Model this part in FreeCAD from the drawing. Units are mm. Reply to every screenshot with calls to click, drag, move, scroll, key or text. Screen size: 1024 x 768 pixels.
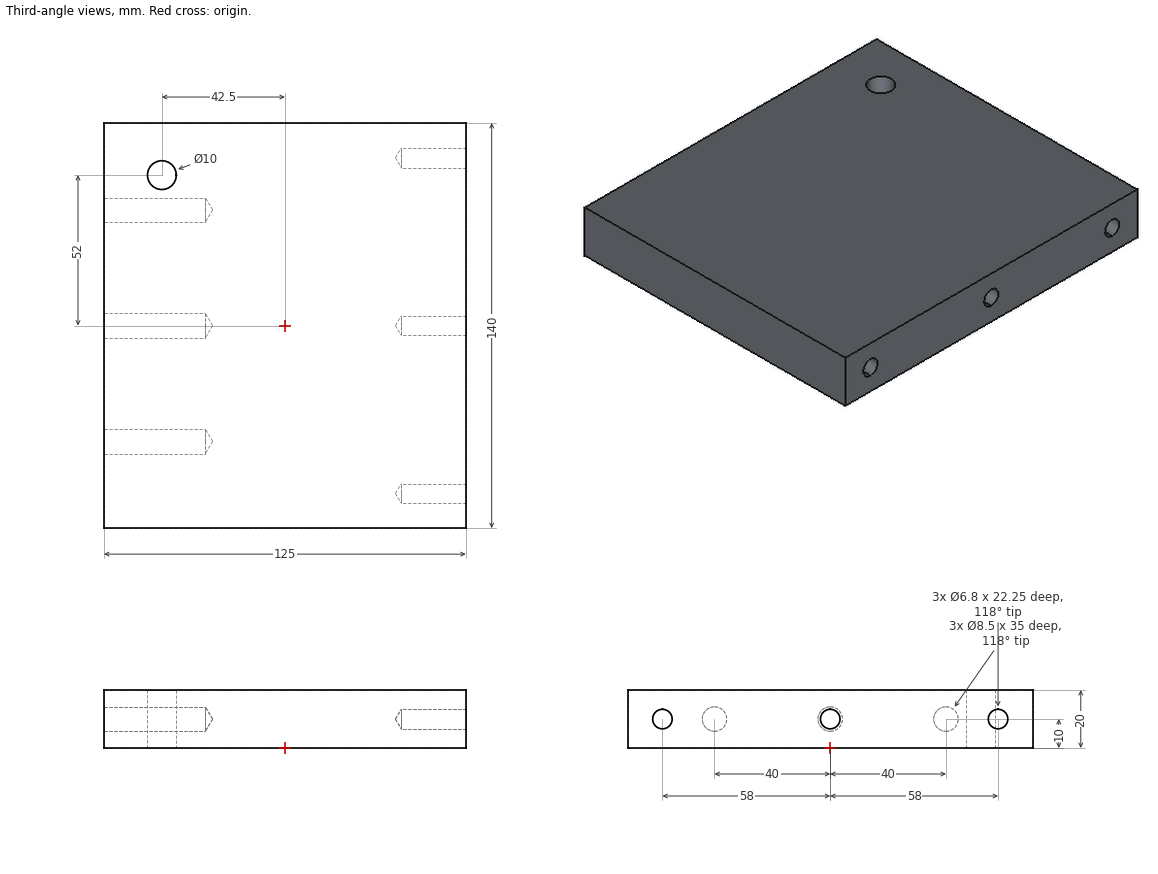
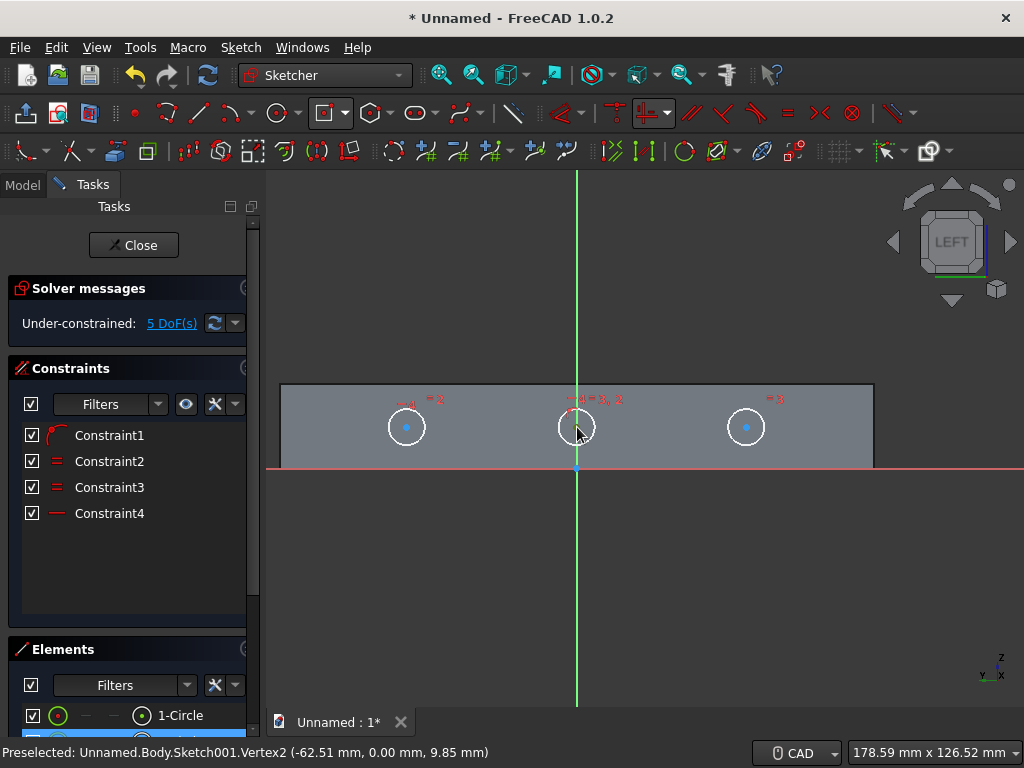
click(746, 427)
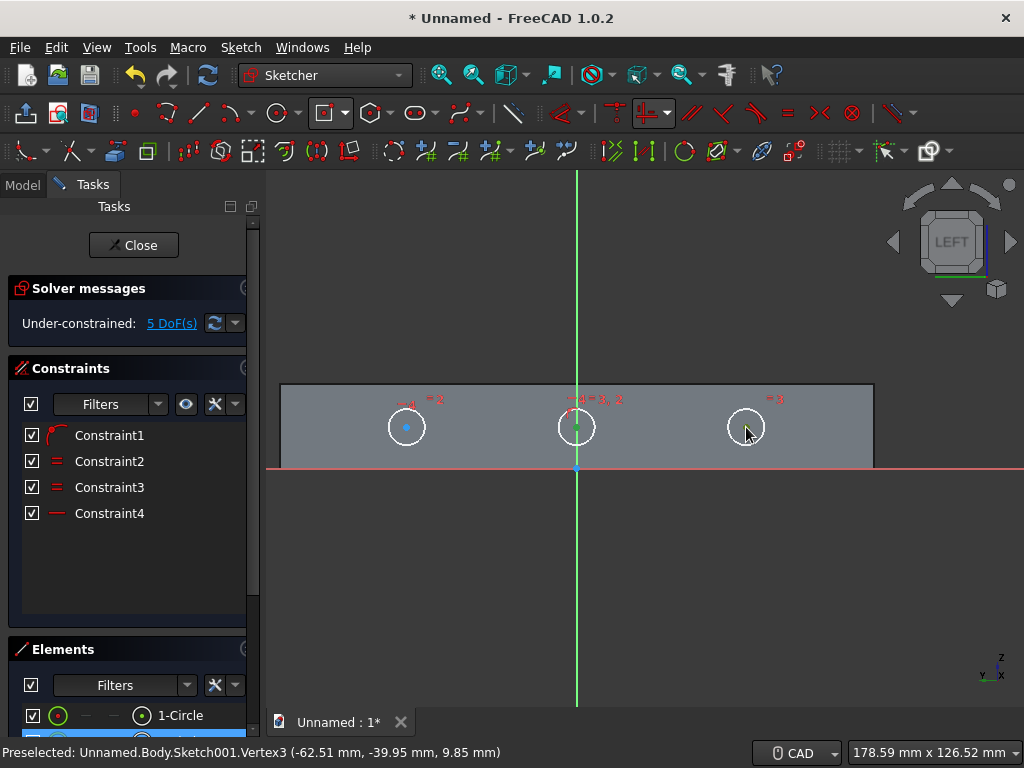
click(670, 114)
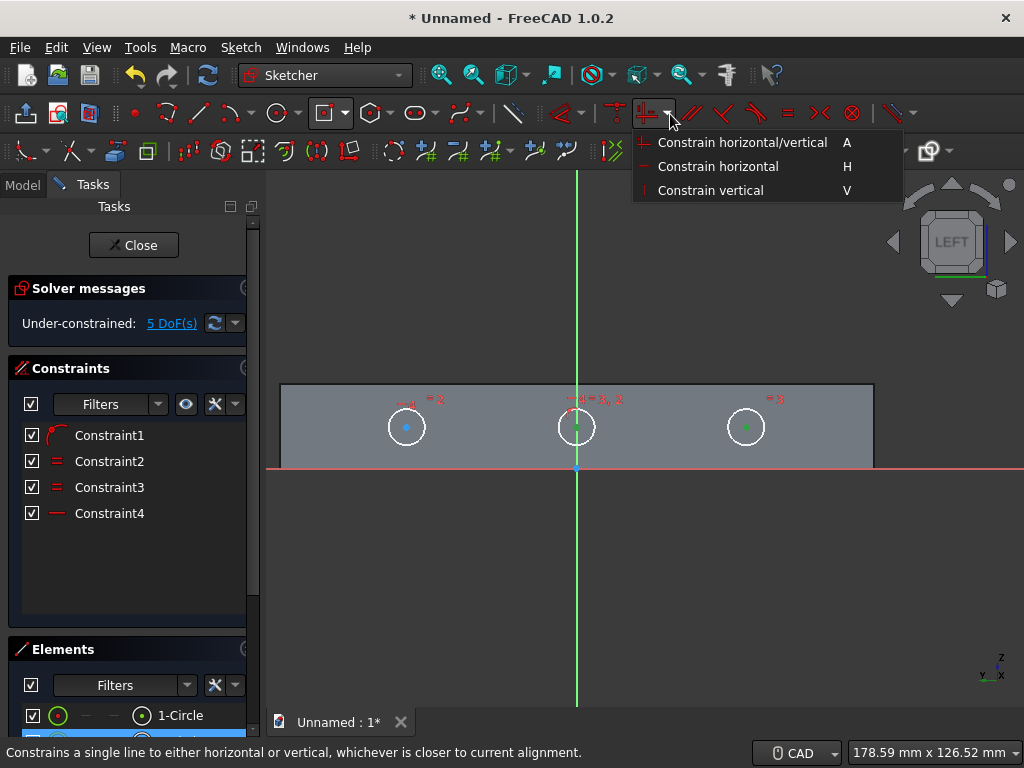
click(768, 166)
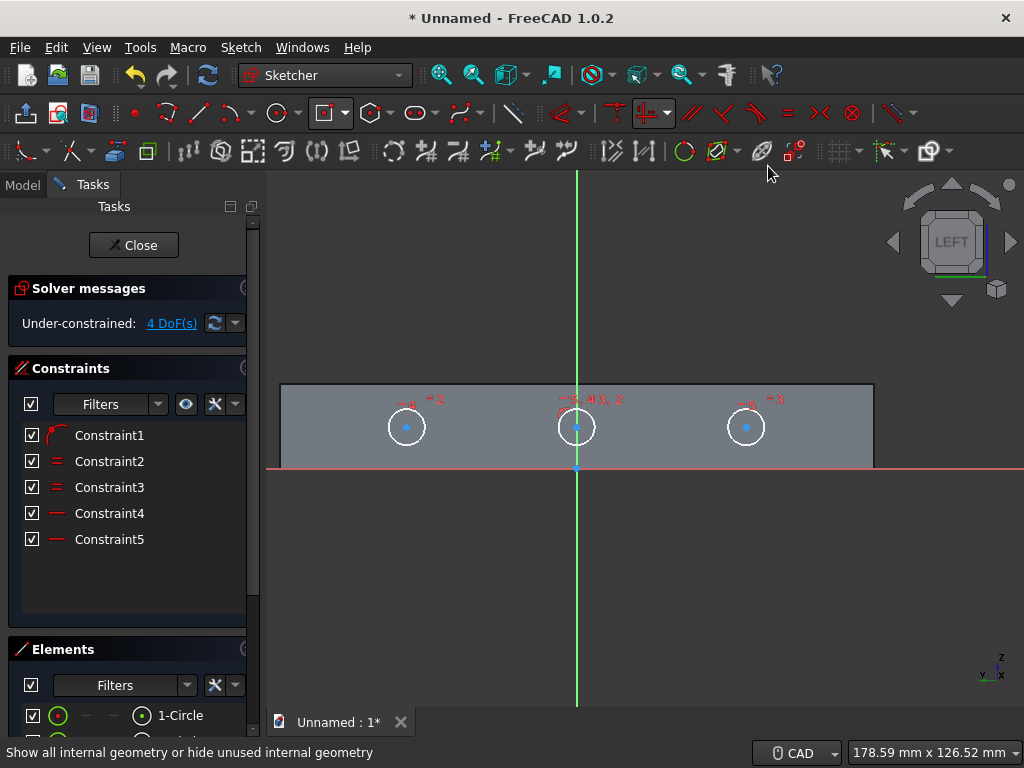
click(560, 114)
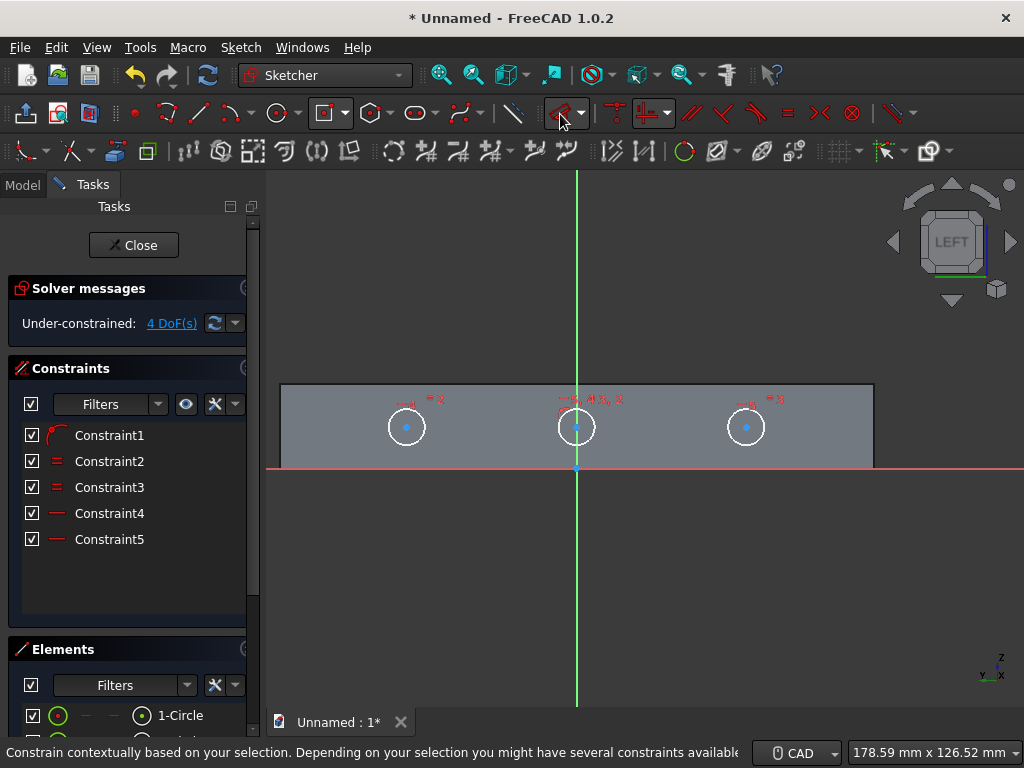
click(419, 414)
click(441, 391)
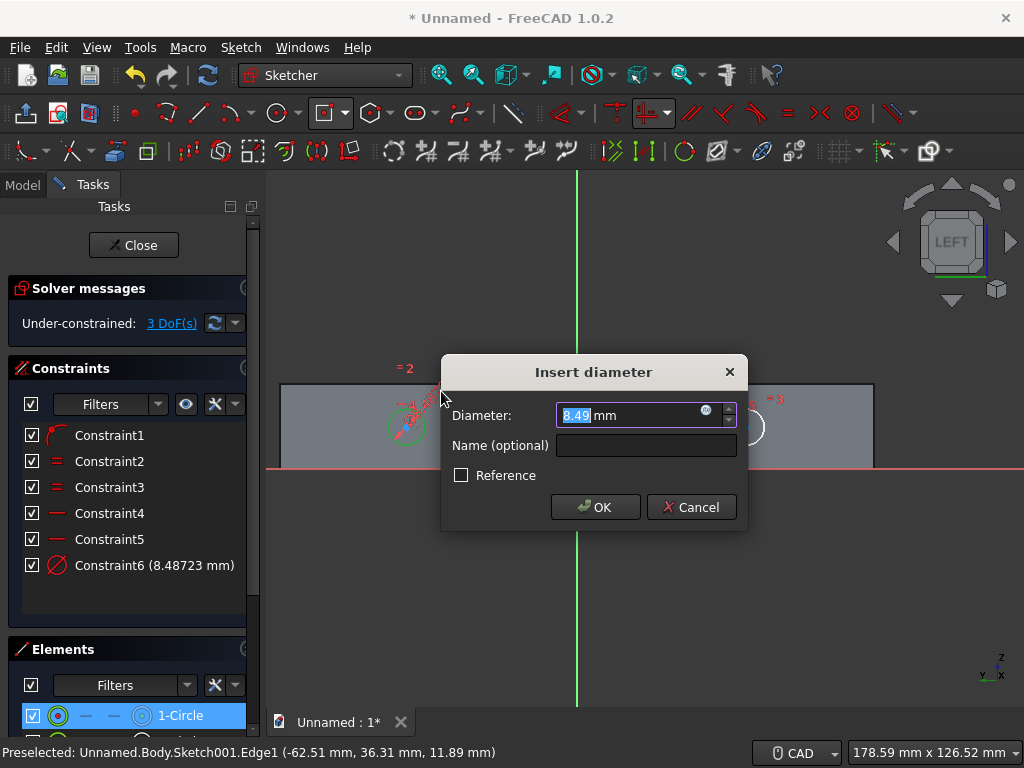
text(8.5)
key(Return)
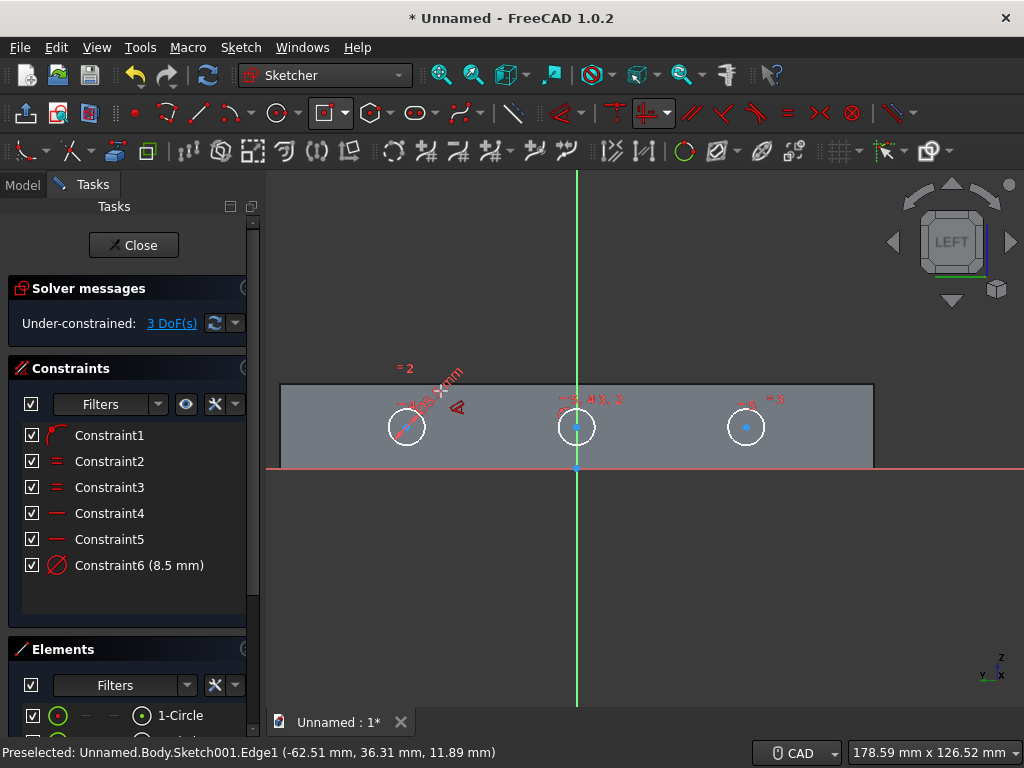
click(407, 427)
click(492, 503)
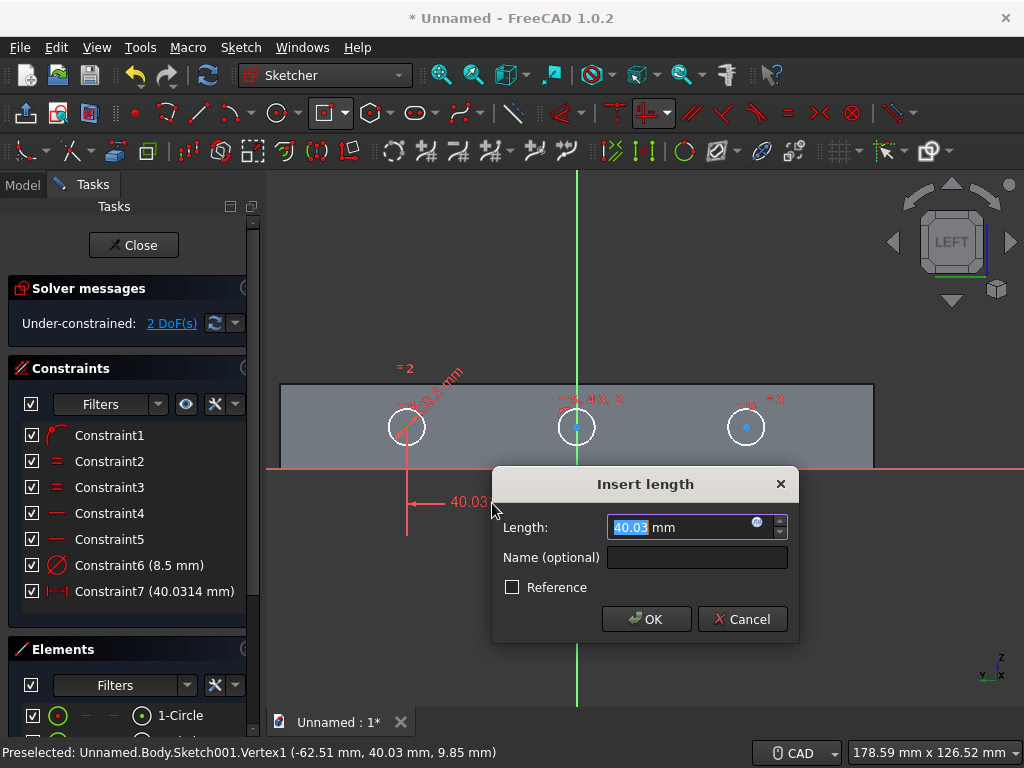
text(40)
key(Return)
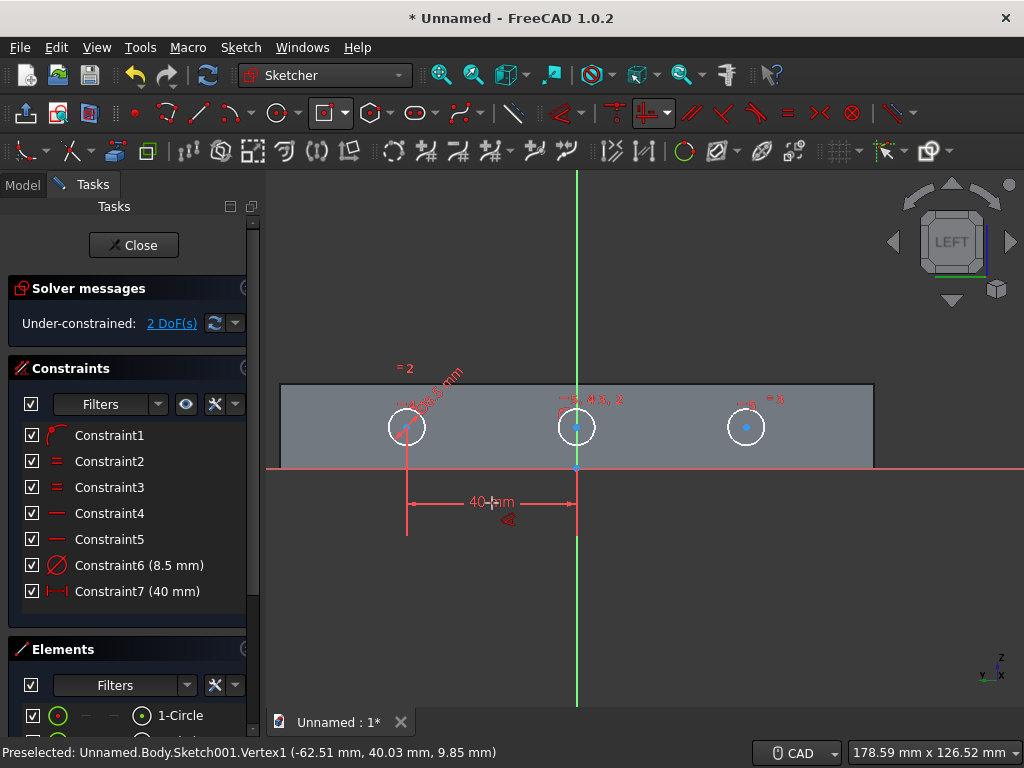
click(407, 427)
click(373, 448)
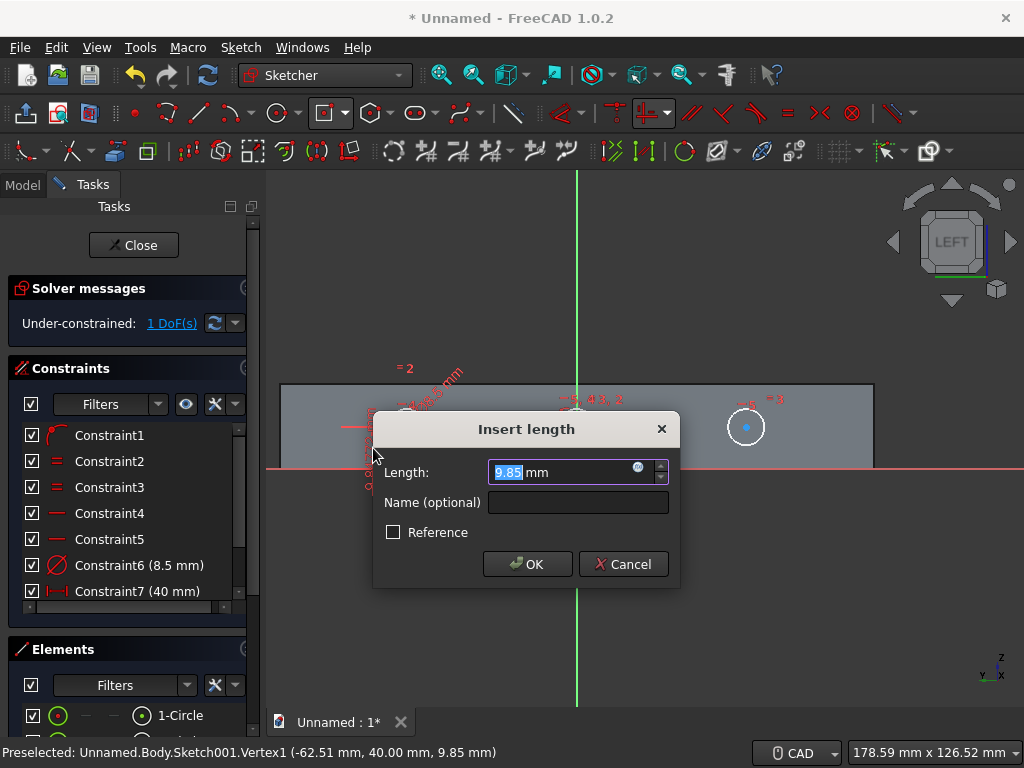
text(10)
key(Return)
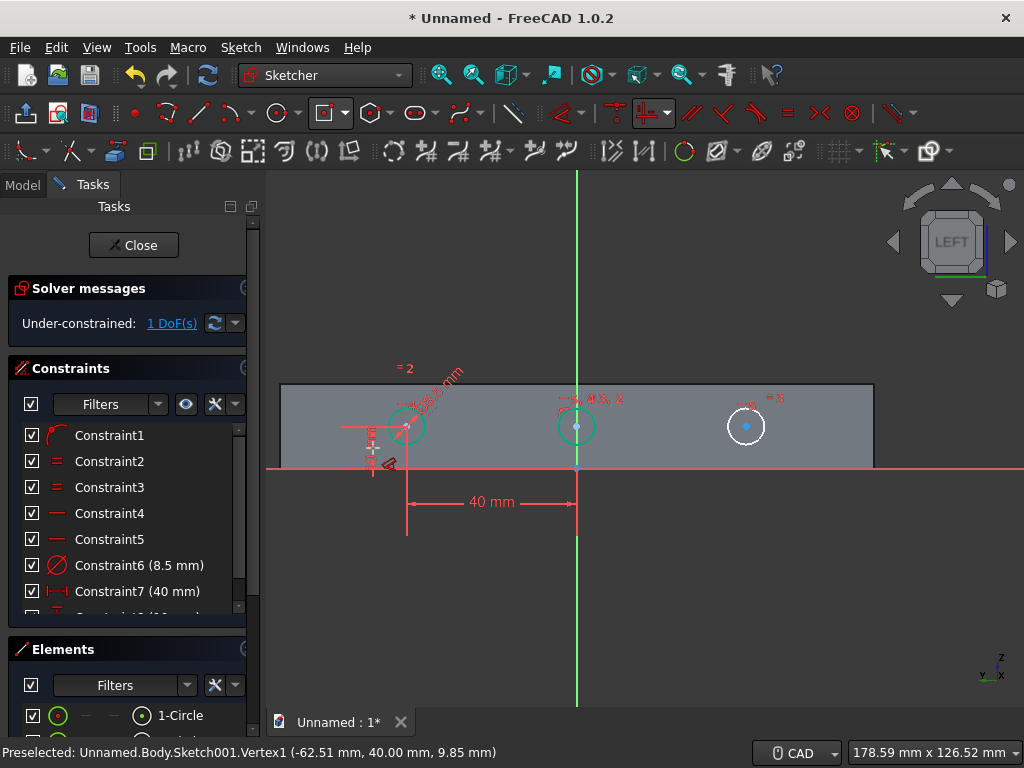
click(746, 427)
click(661, 503)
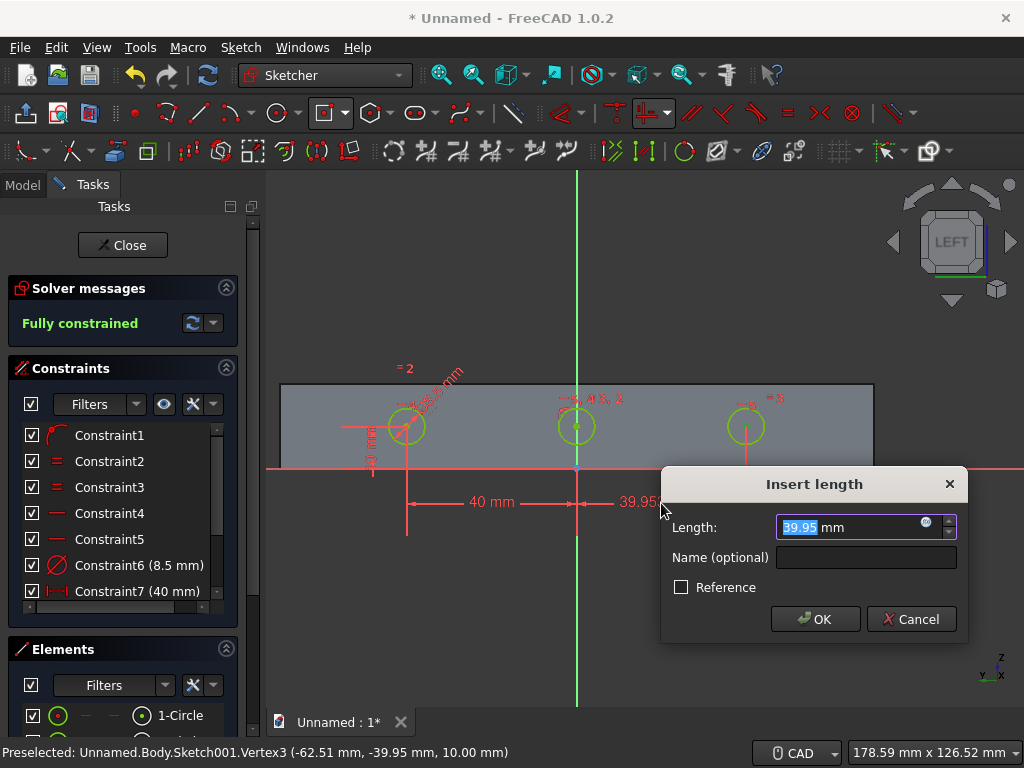
text(40)
key(Return)
key(Escape)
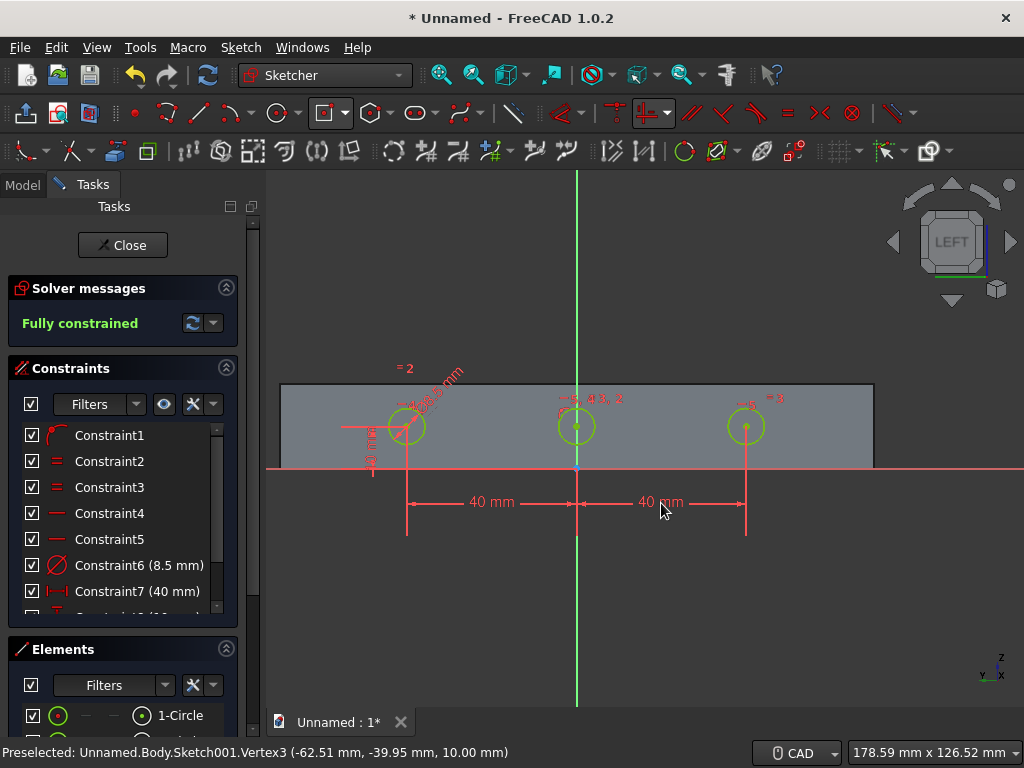
click(123, 245)